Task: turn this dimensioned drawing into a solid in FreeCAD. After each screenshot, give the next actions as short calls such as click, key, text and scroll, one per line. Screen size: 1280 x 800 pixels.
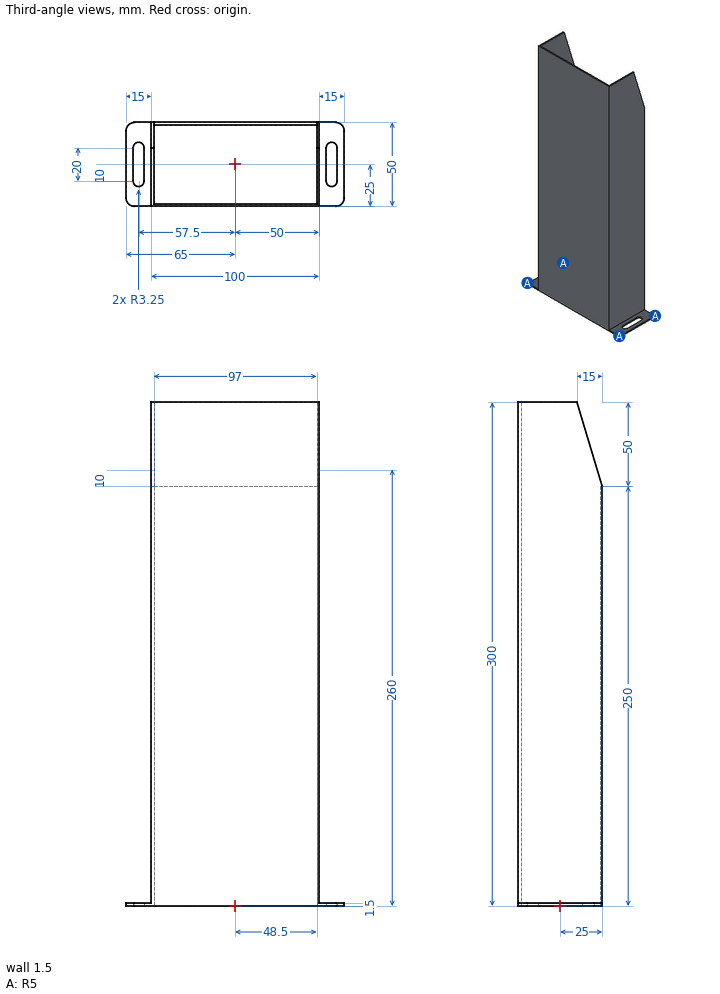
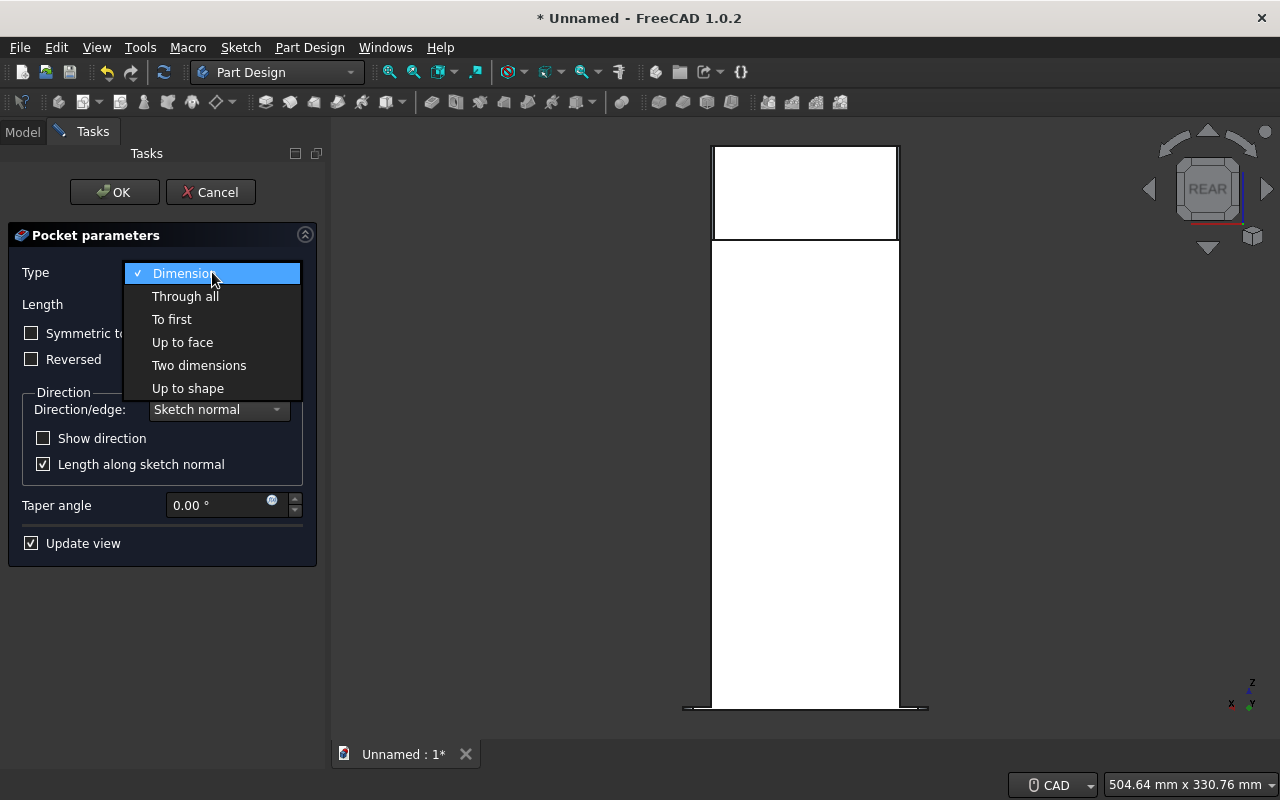
click(212, 320)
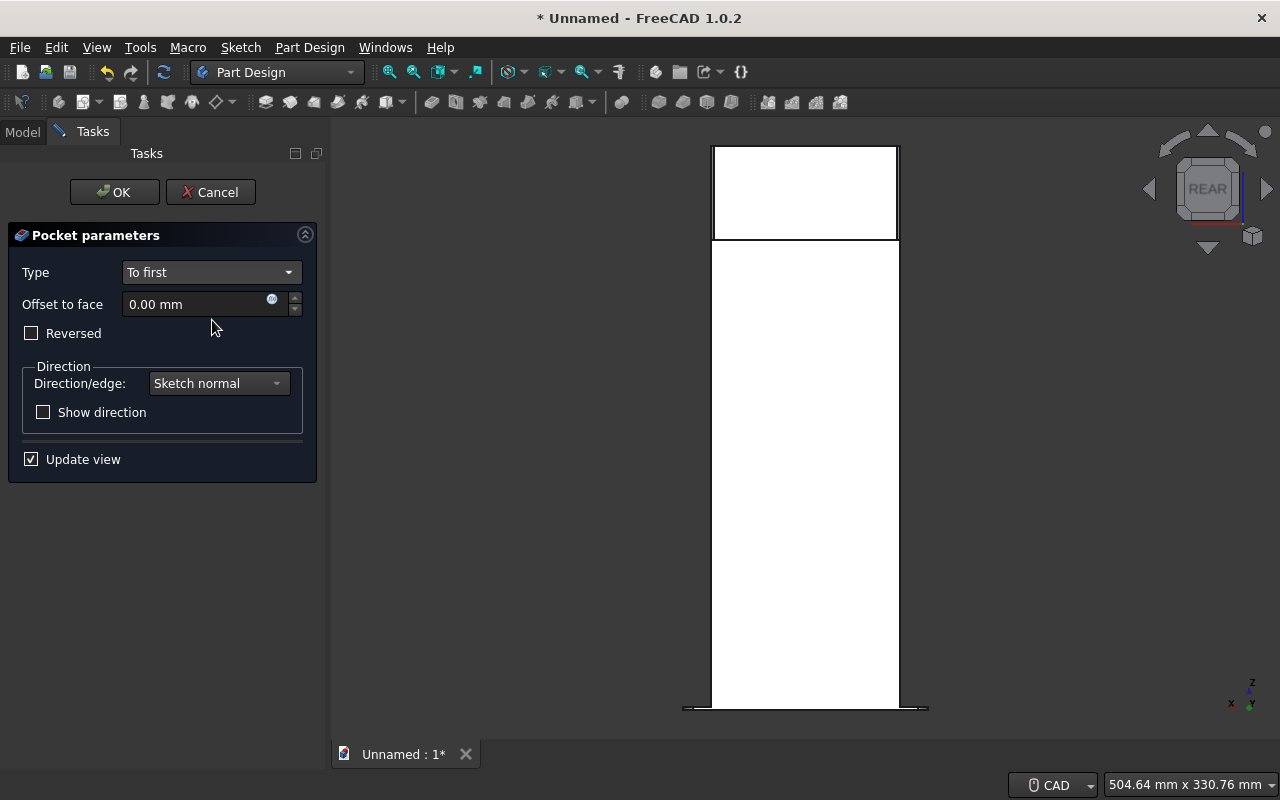
click(115, 192)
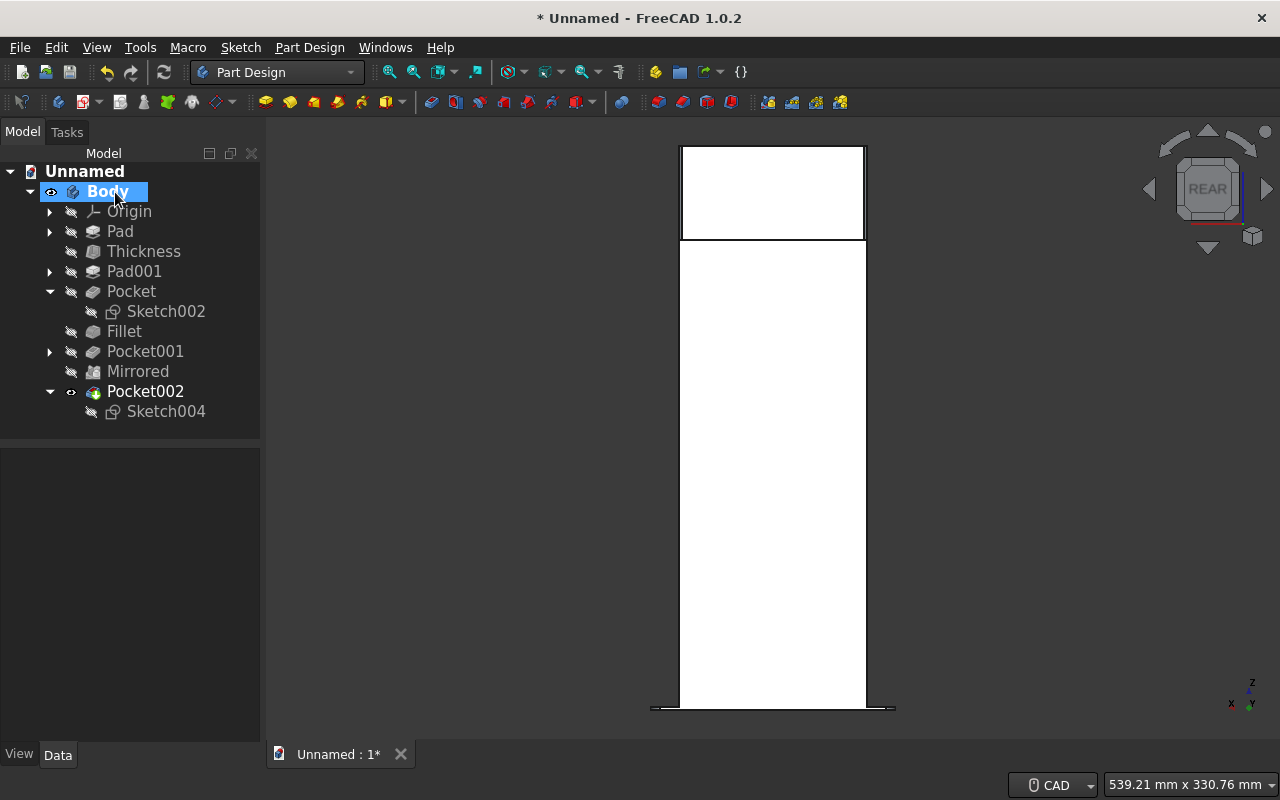
key(0)